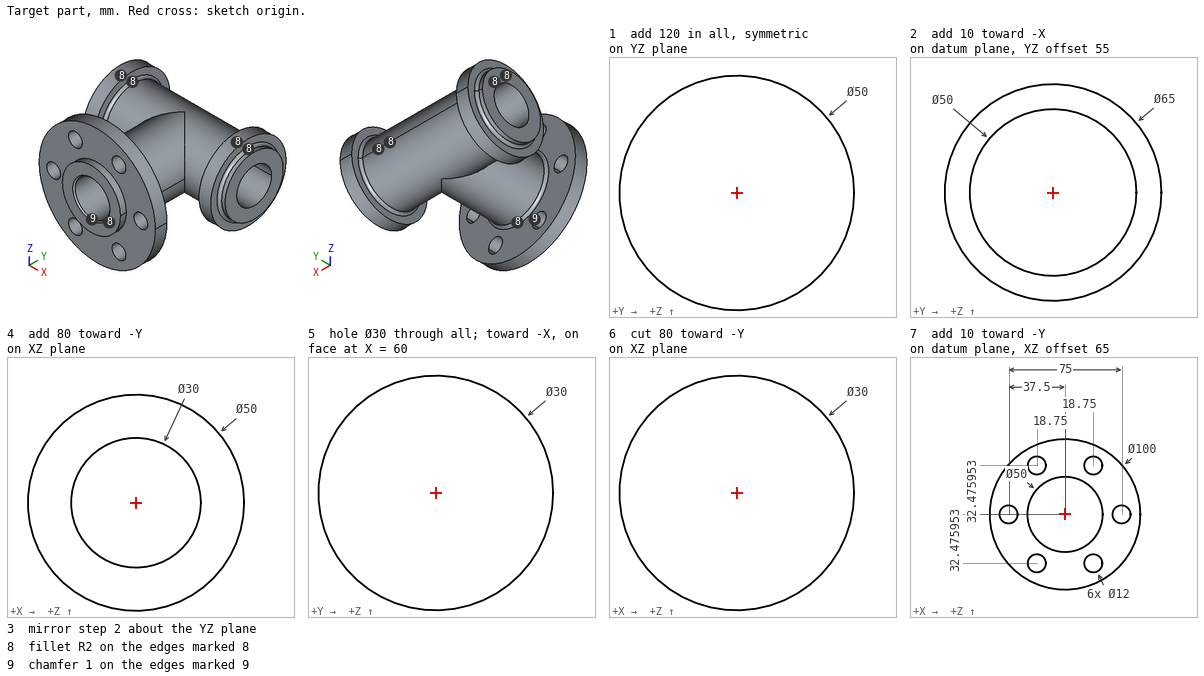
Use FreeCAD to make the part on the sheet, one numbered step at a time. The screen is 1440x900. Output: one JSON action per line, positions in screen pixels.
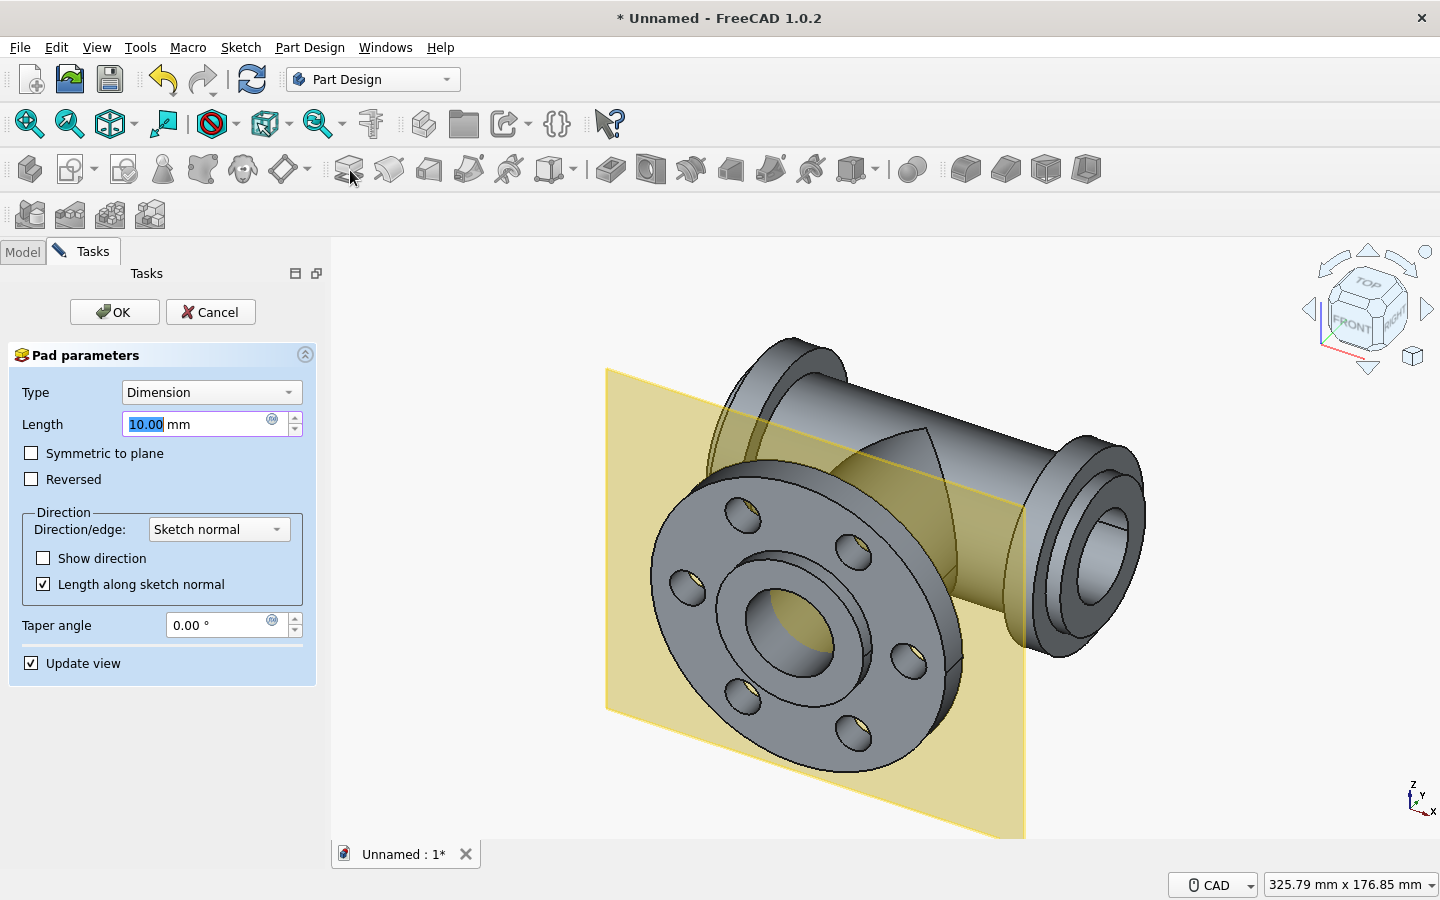
{"action": "type", "text": "10"}
{"action": "key", "text": "Tab"}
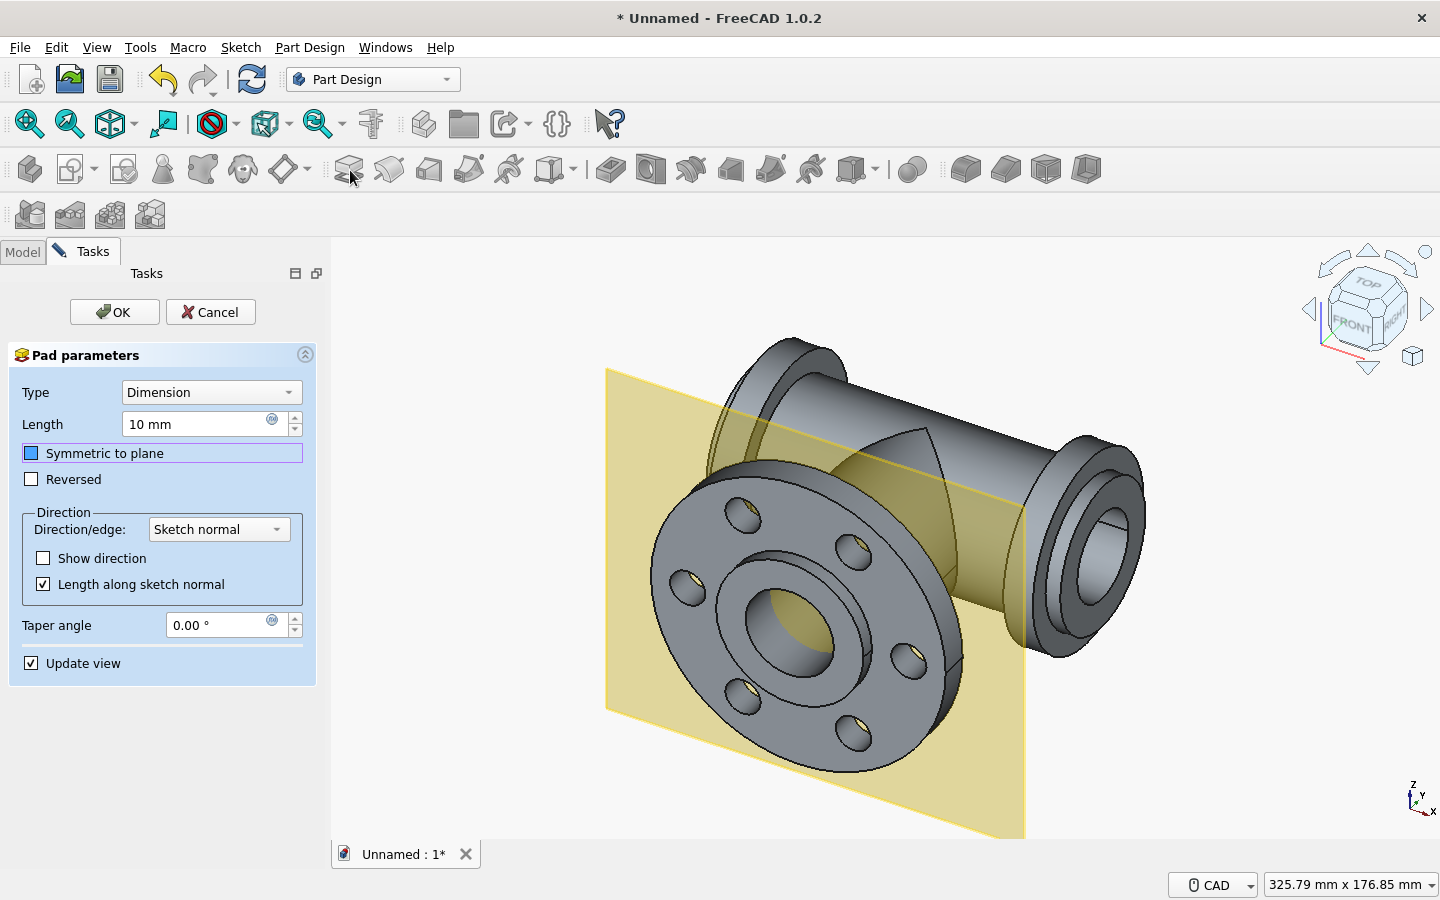
{"action": "left_click", "coordinate": [115, 312]}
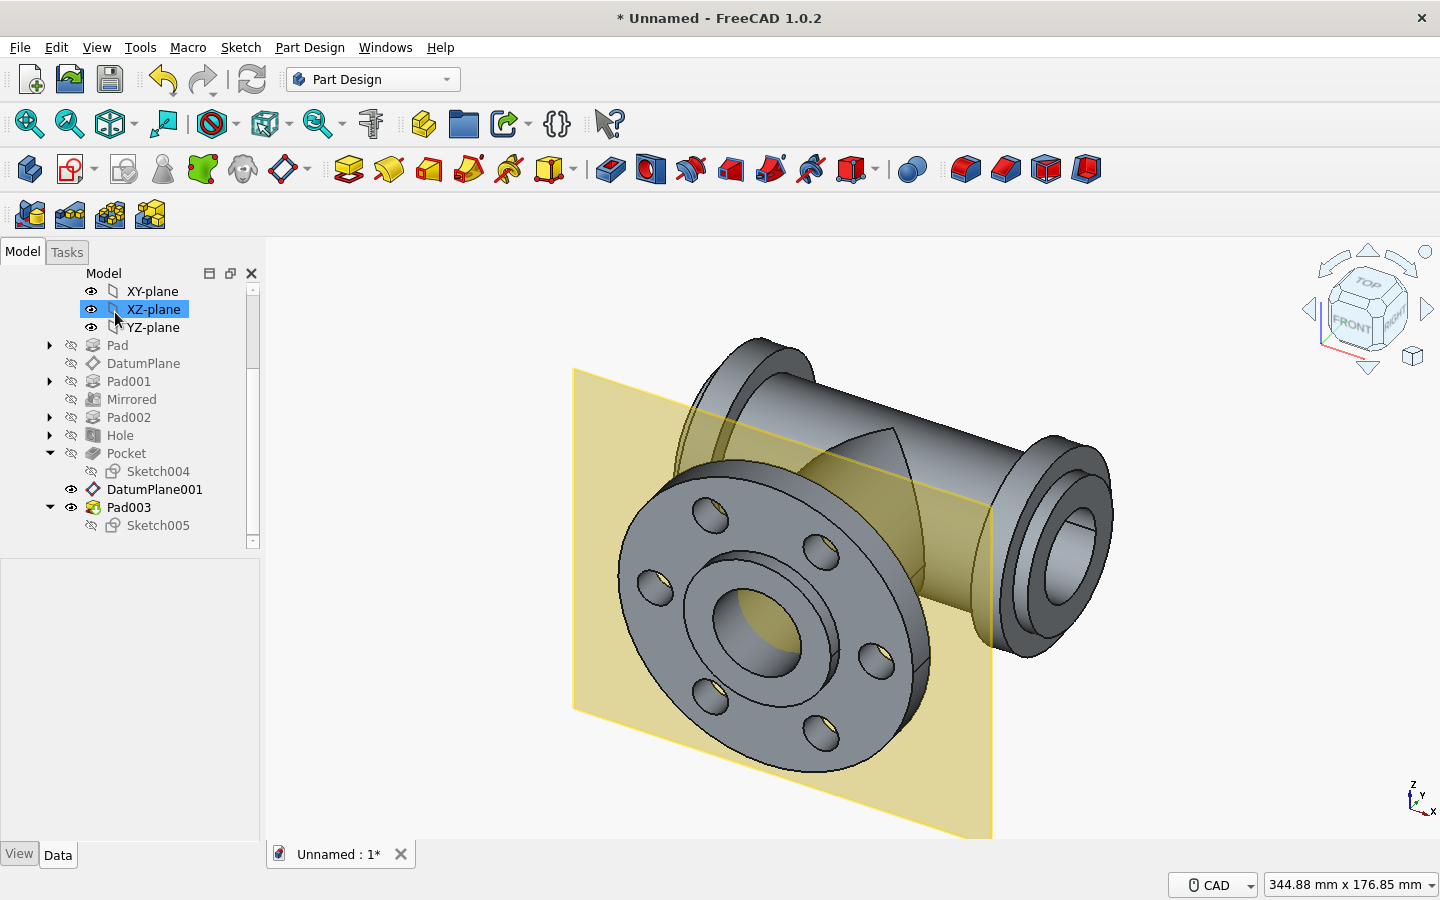
{"action": "left_click", "coordinate": [116, 489]}
{"action": "key", "text": "space"}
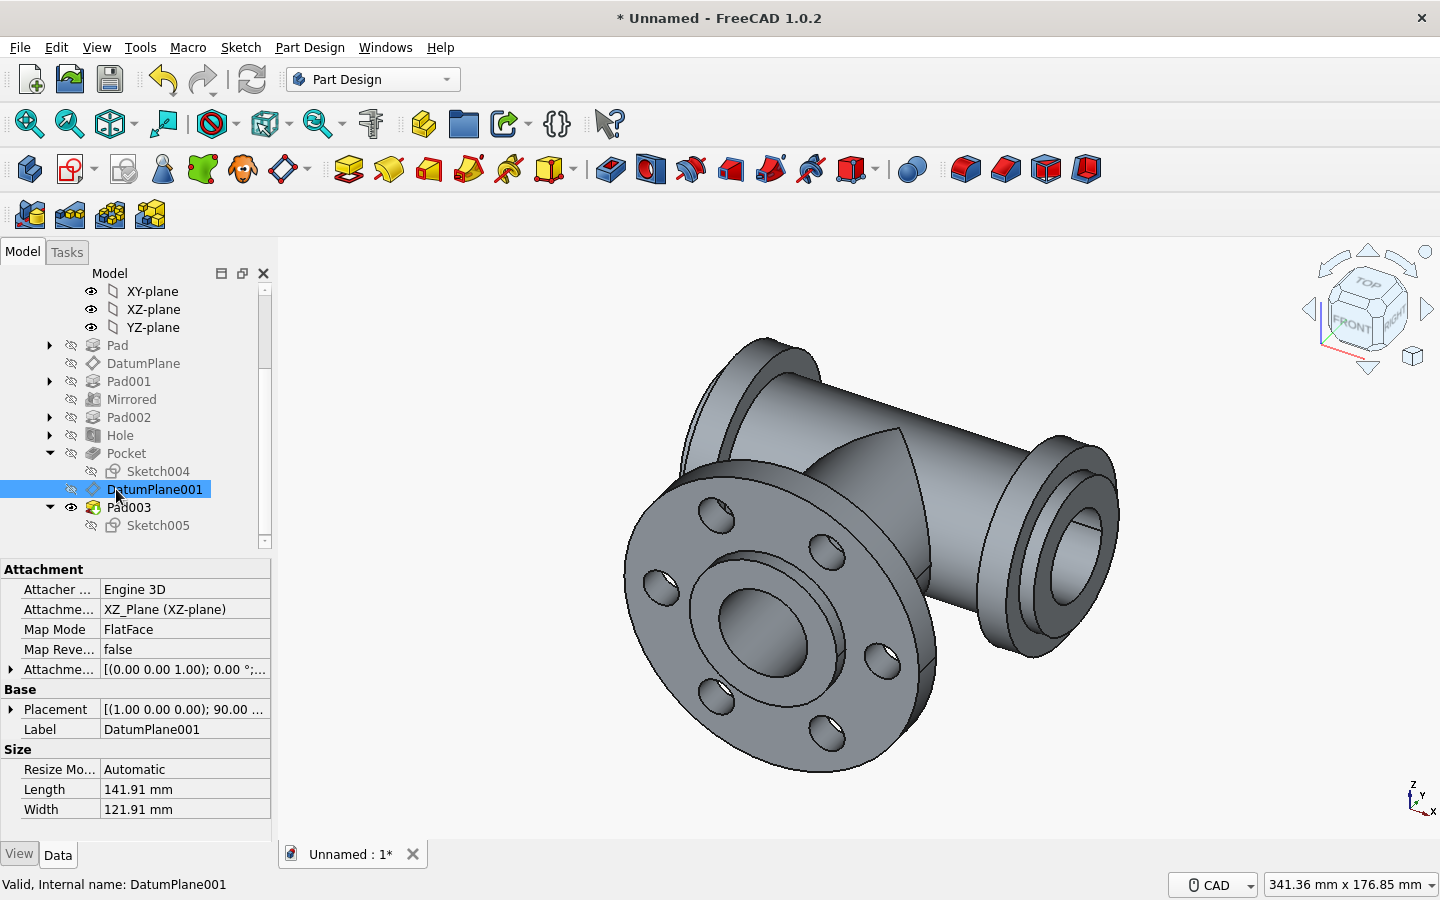
{"action": "key", "text": "0"}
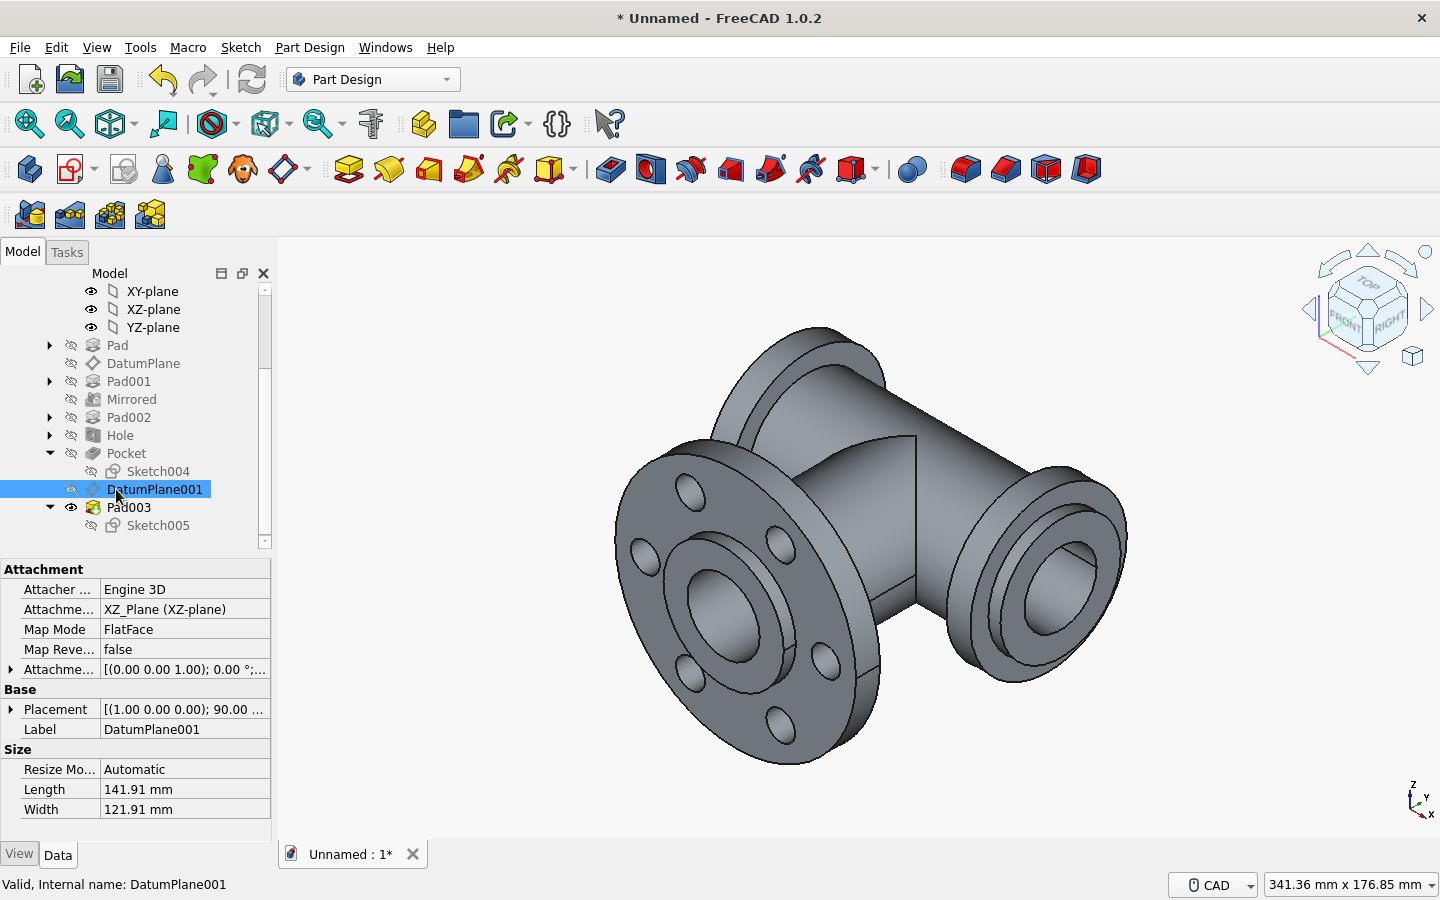
{"action": "key", "text": "v f"}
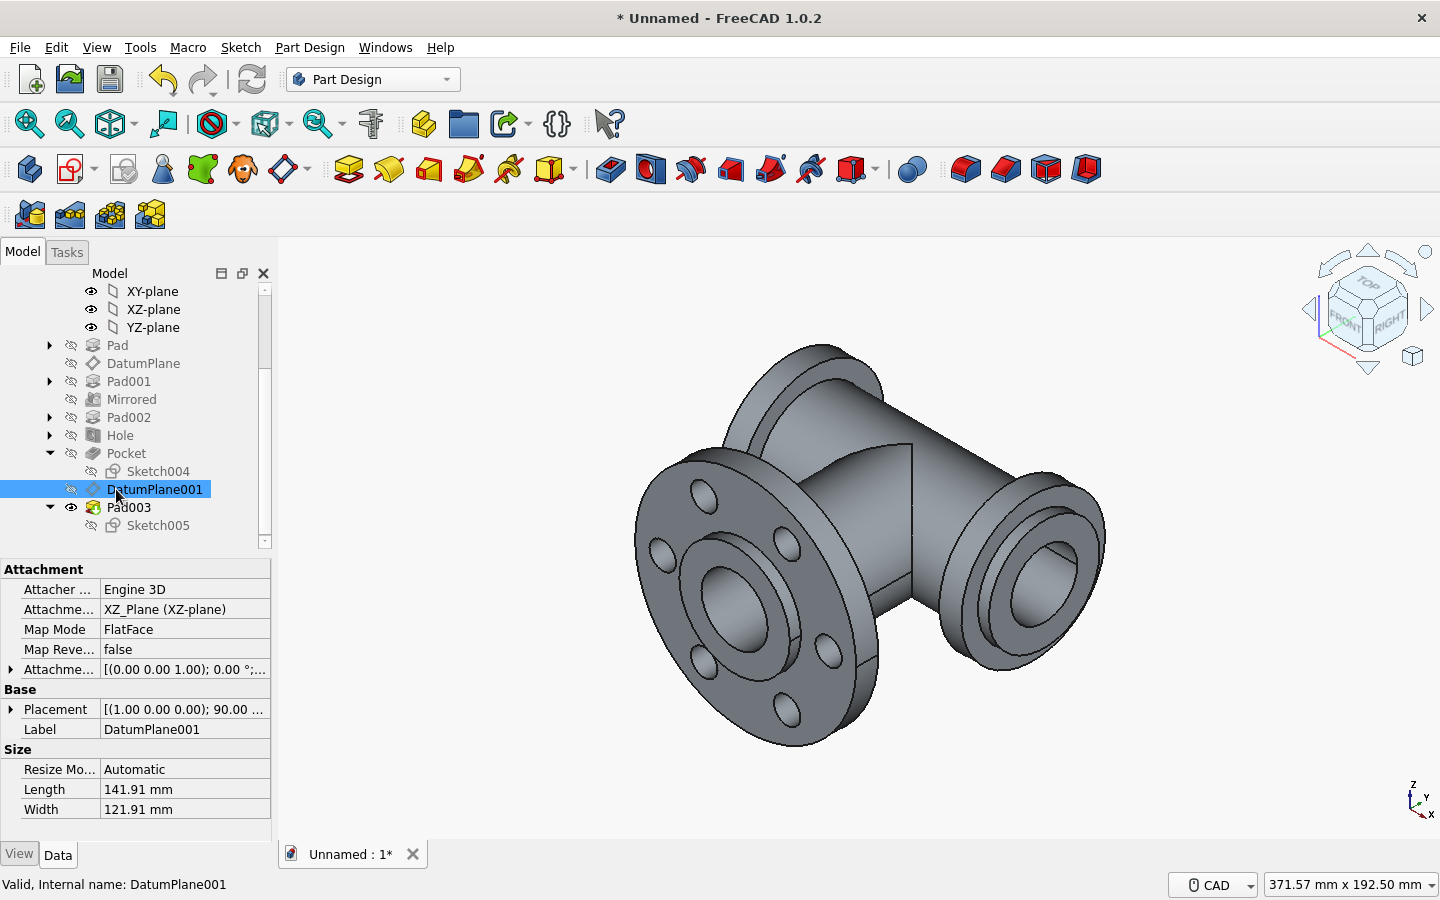
{"action": "key", "text": "2"}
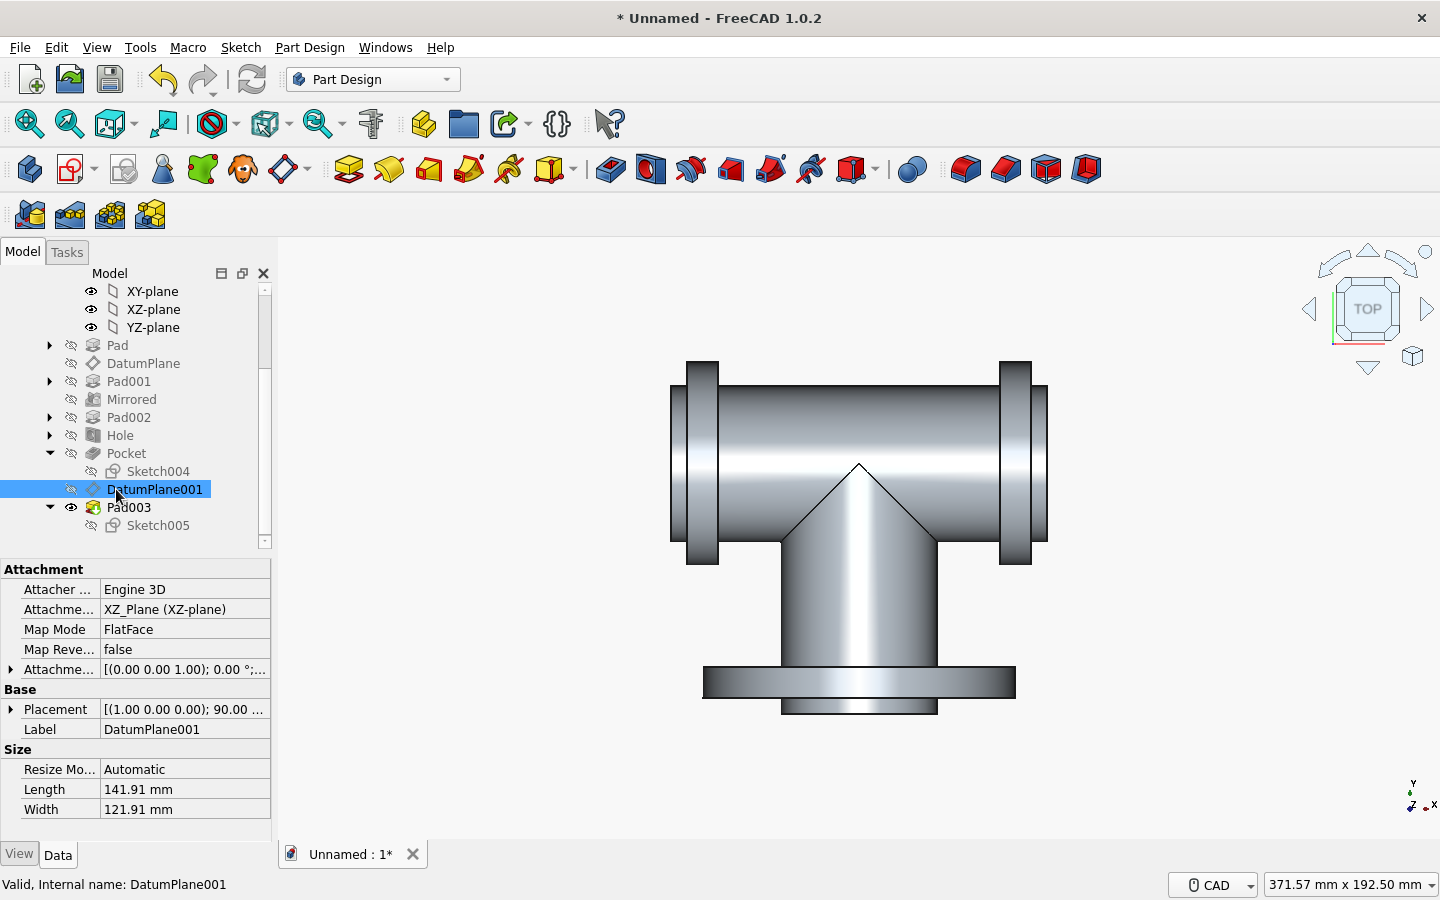
{"action": "key", "text": "1"}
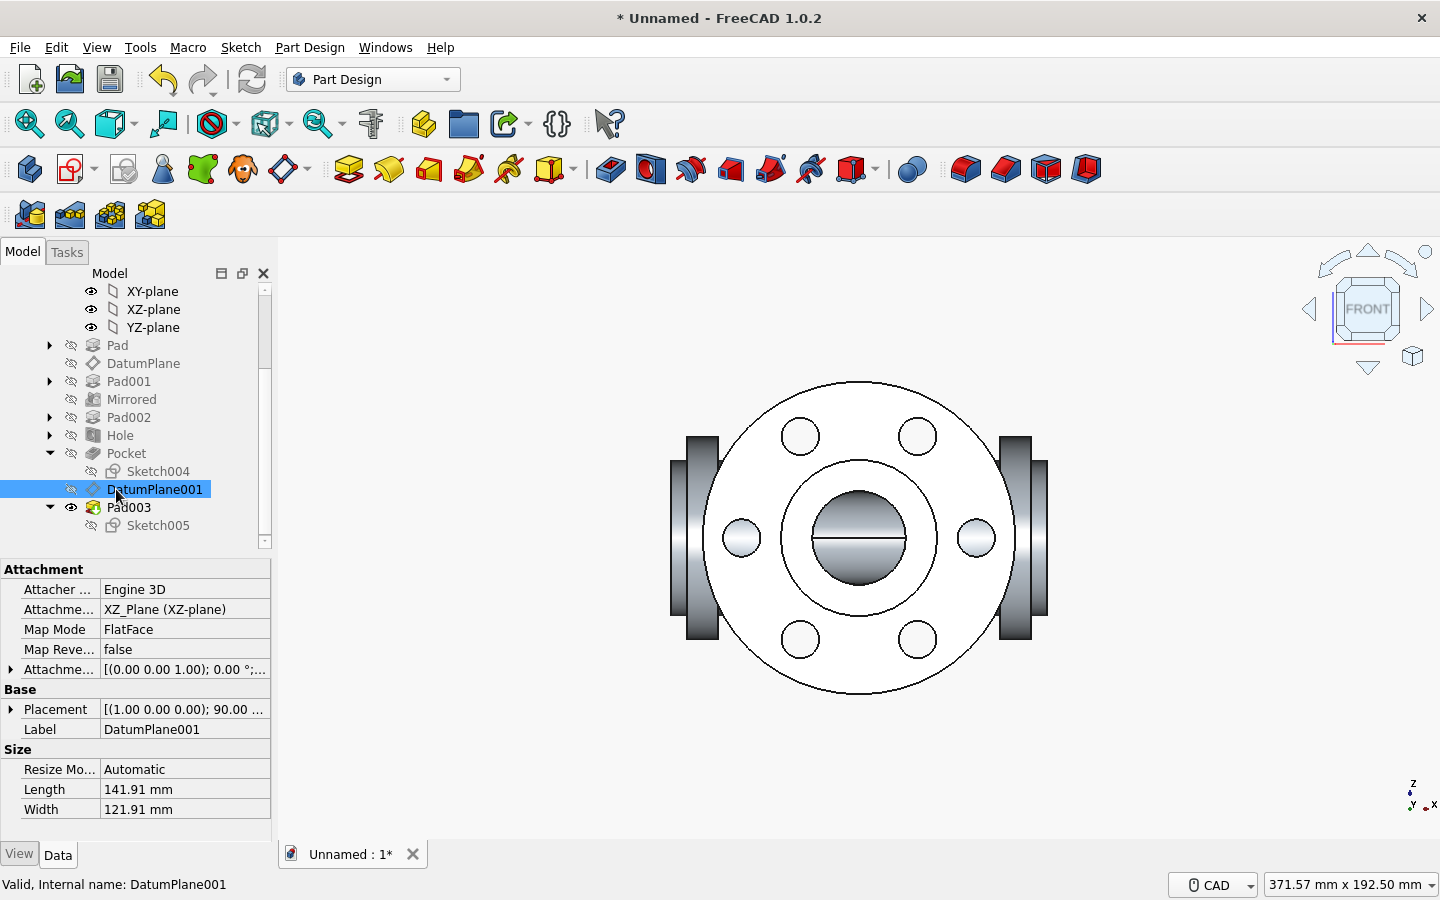
{"action": "key", "text": "3"}